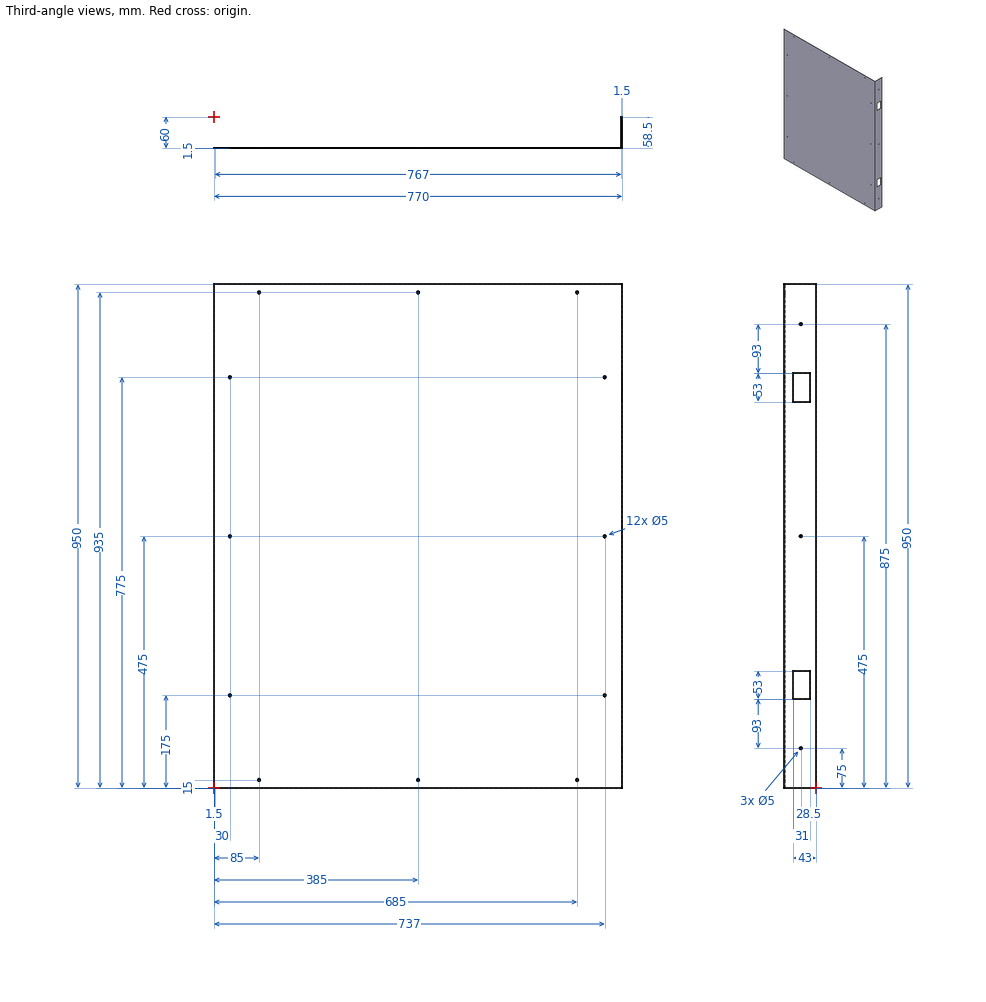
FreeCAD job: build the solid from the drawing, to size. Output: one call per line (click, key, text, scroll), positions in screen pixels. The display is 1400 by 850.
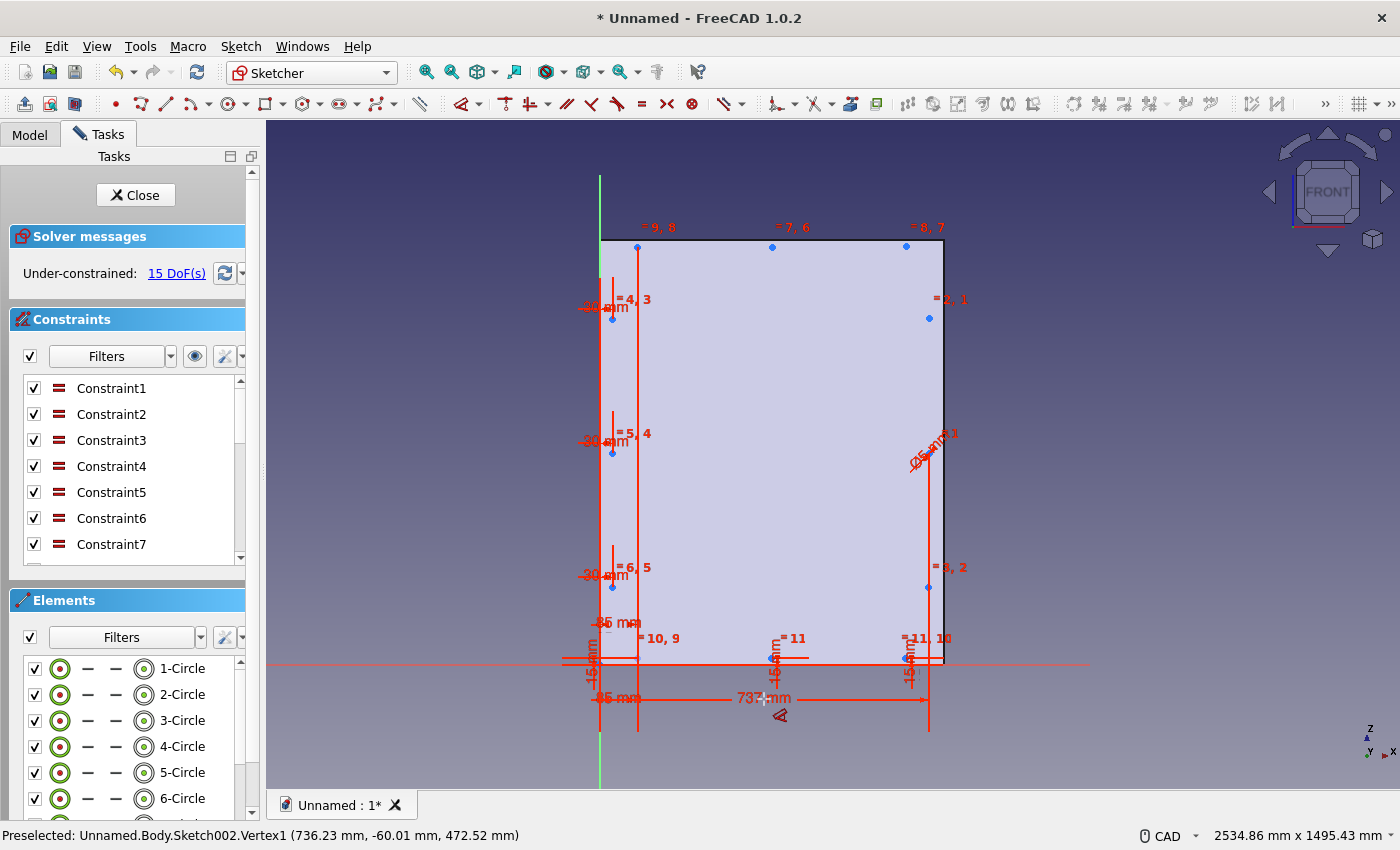
click(929, 453)
click(566, 510)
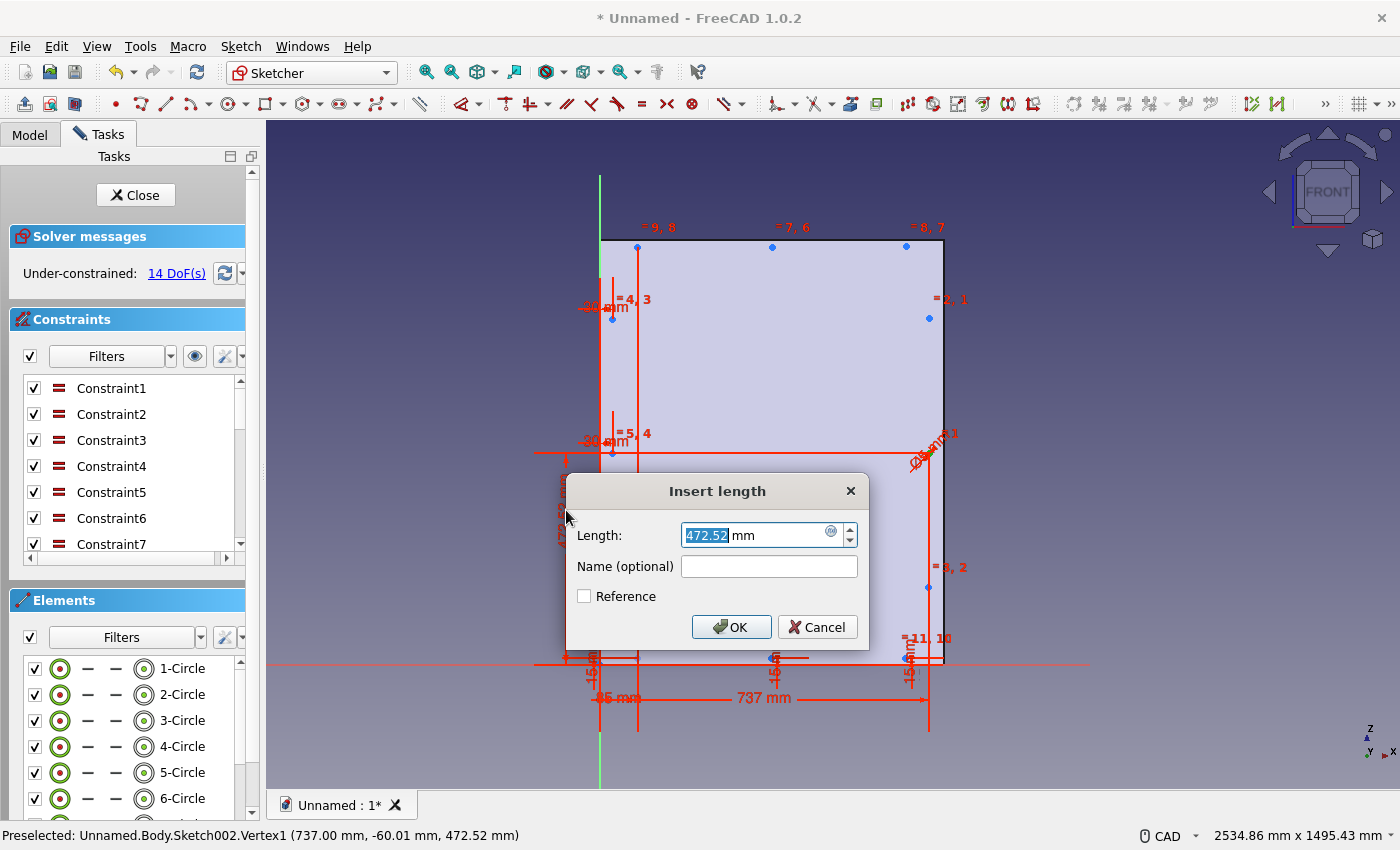
text(475)
key(Return)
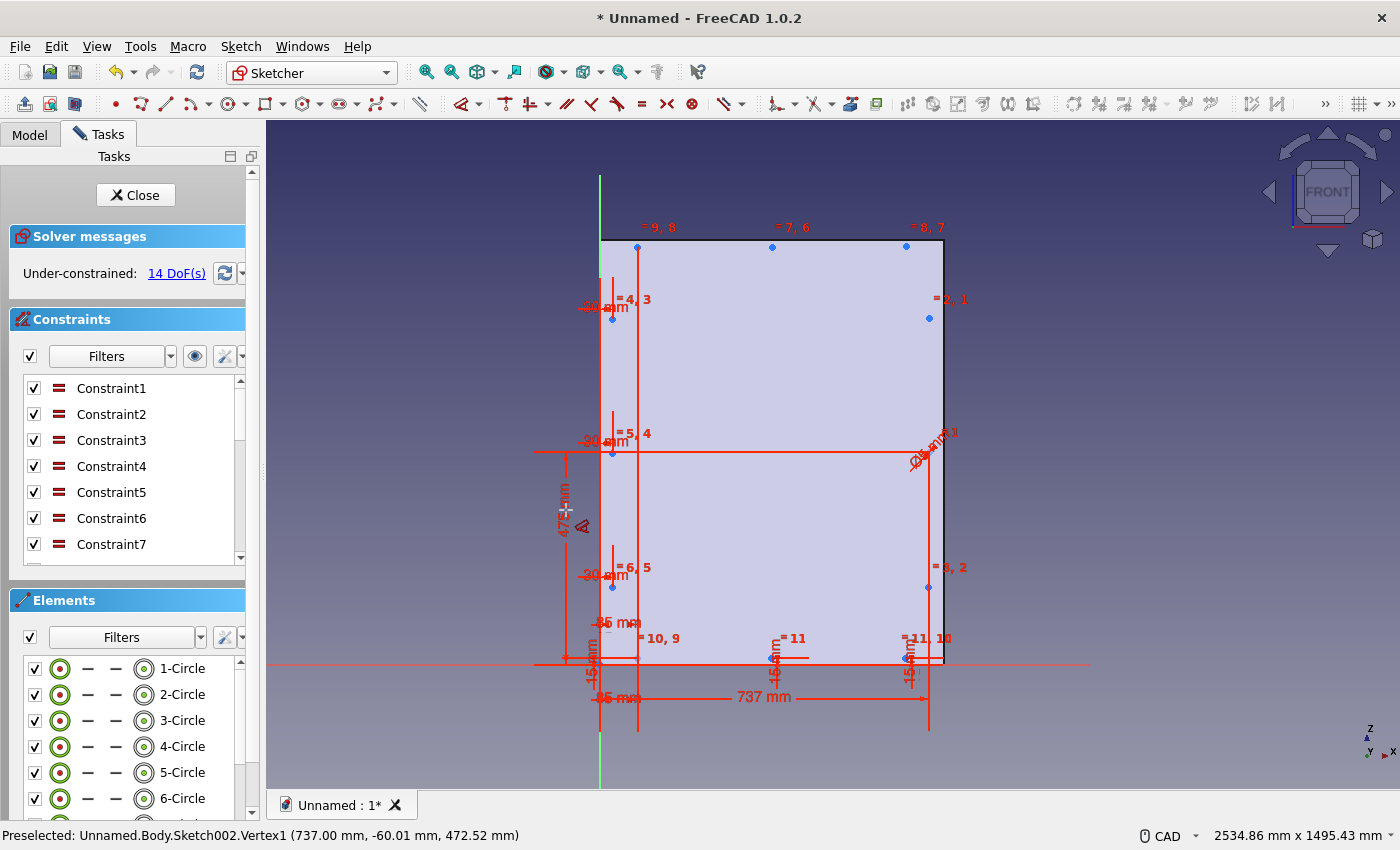
click(929, 319)
click(840, 699)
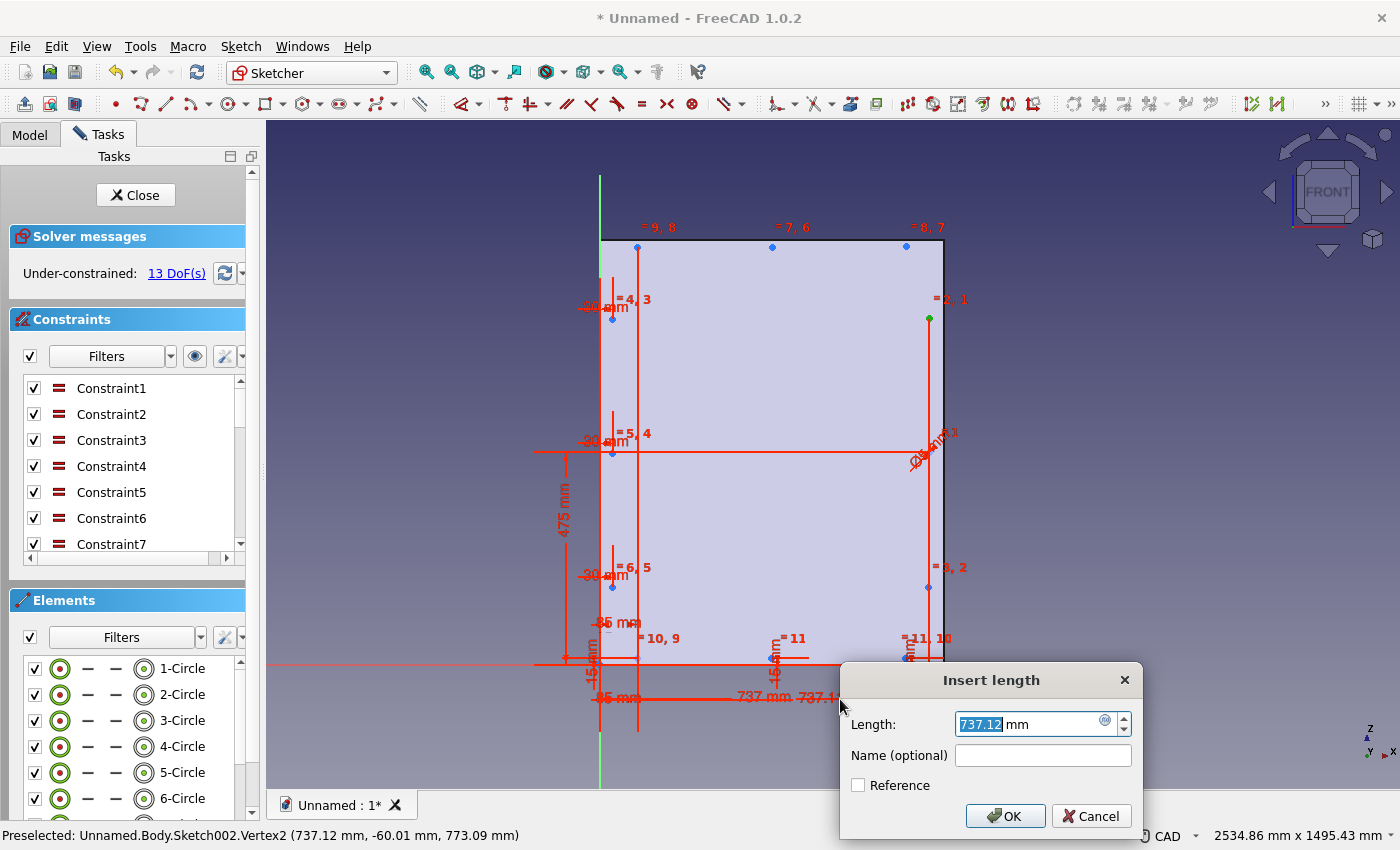
text(737)
key(Return)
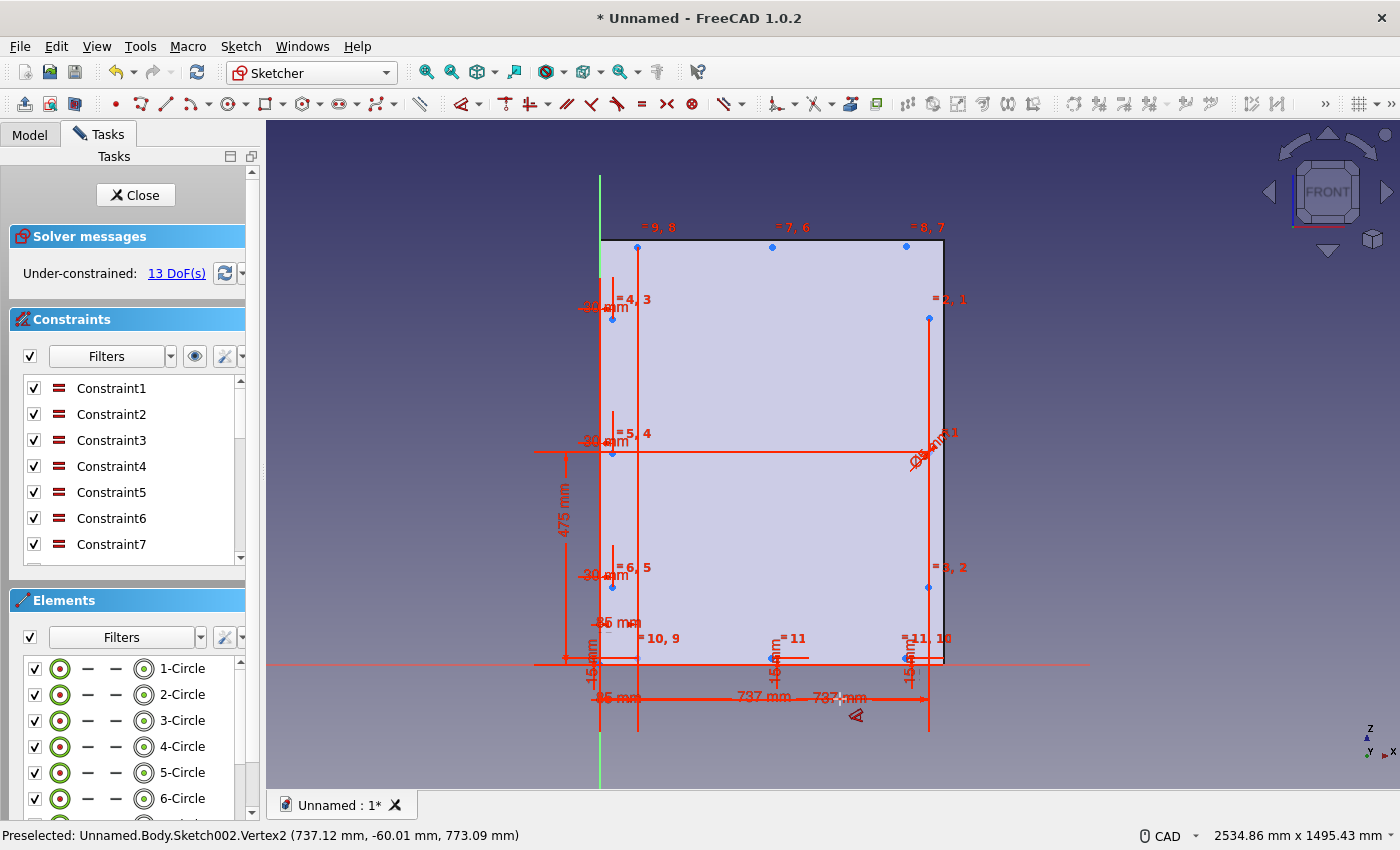
click(929, 319)
click(566, 412)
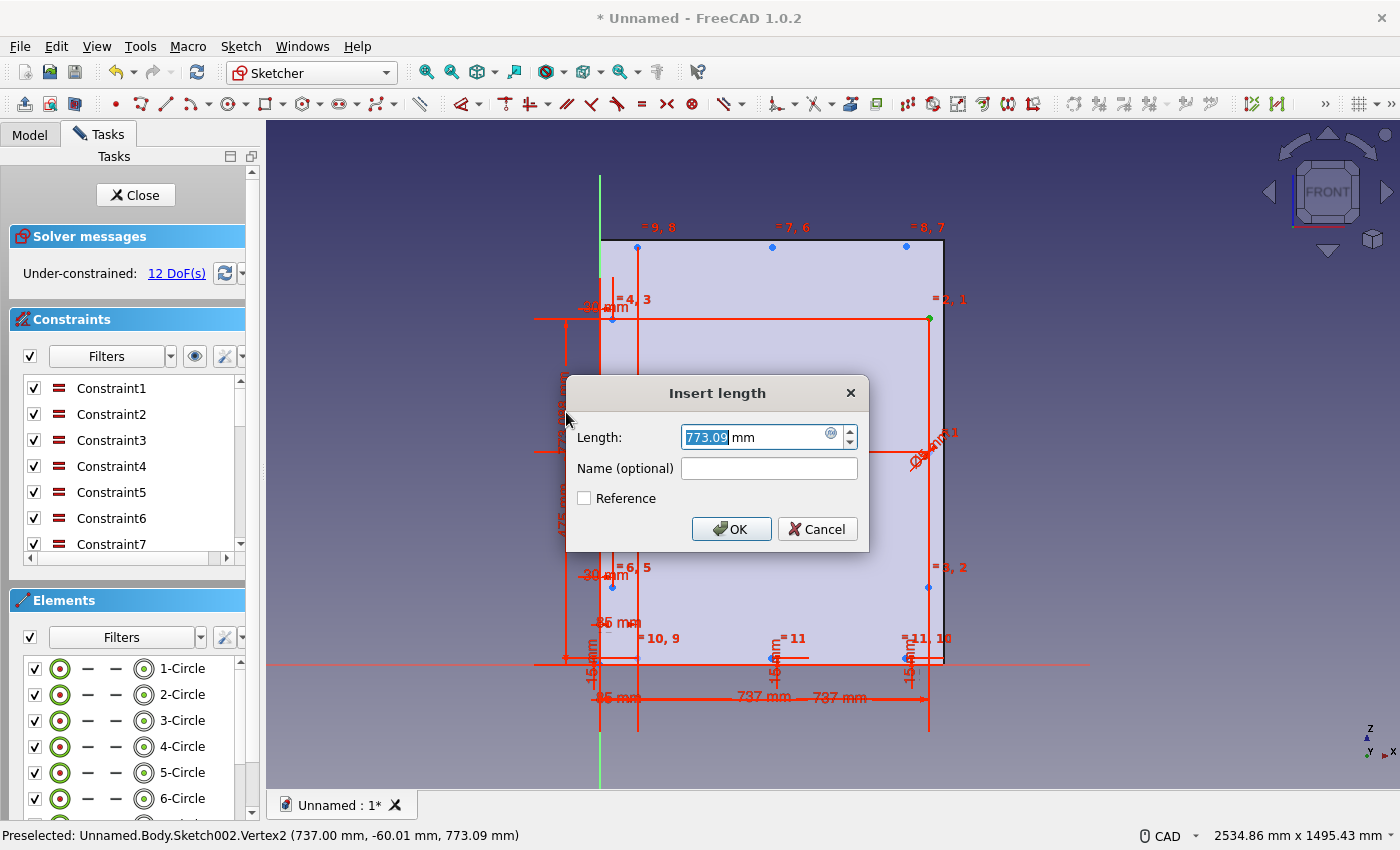
text(775)
key(Return)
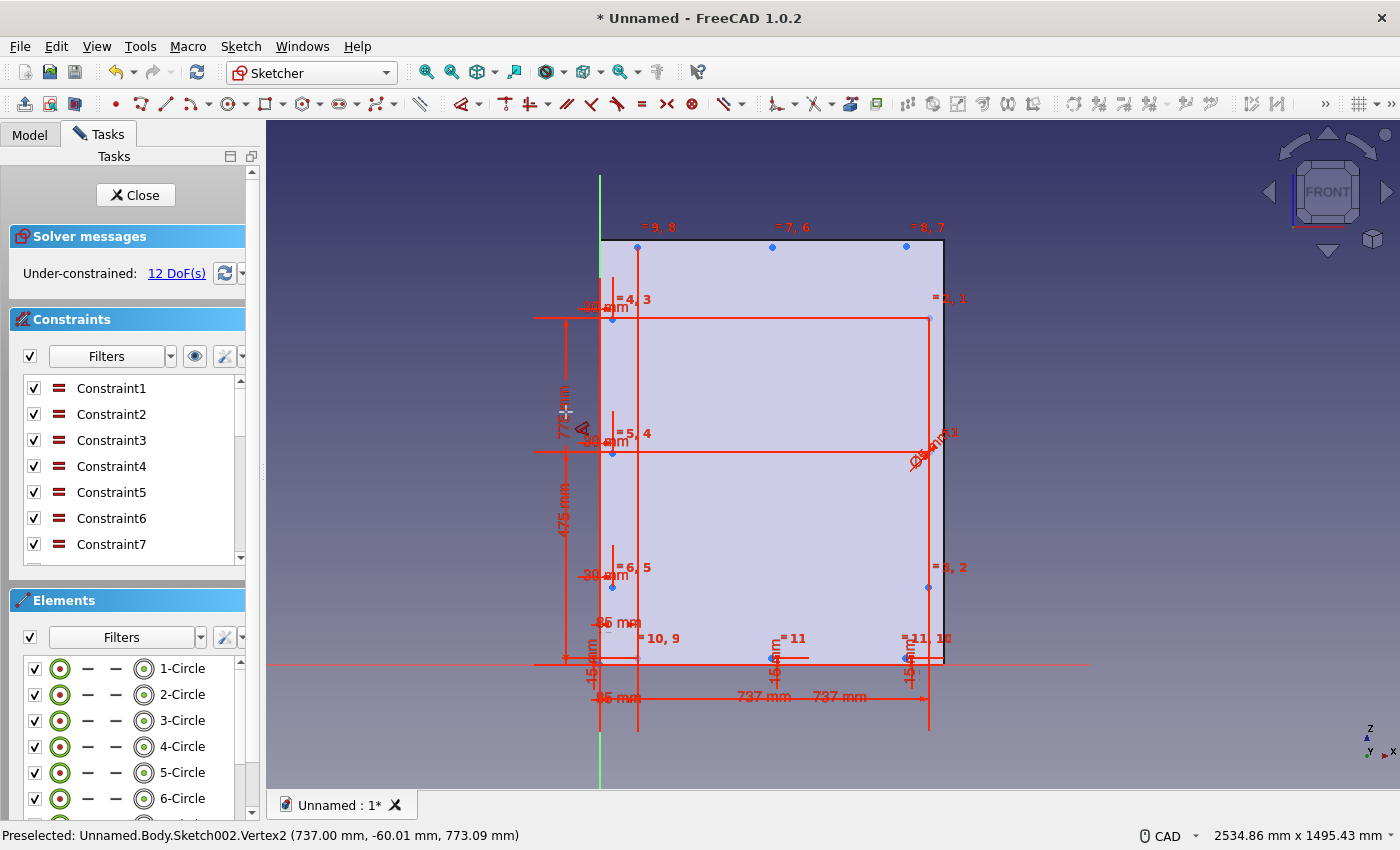
click(929, 588)
click(764, 554)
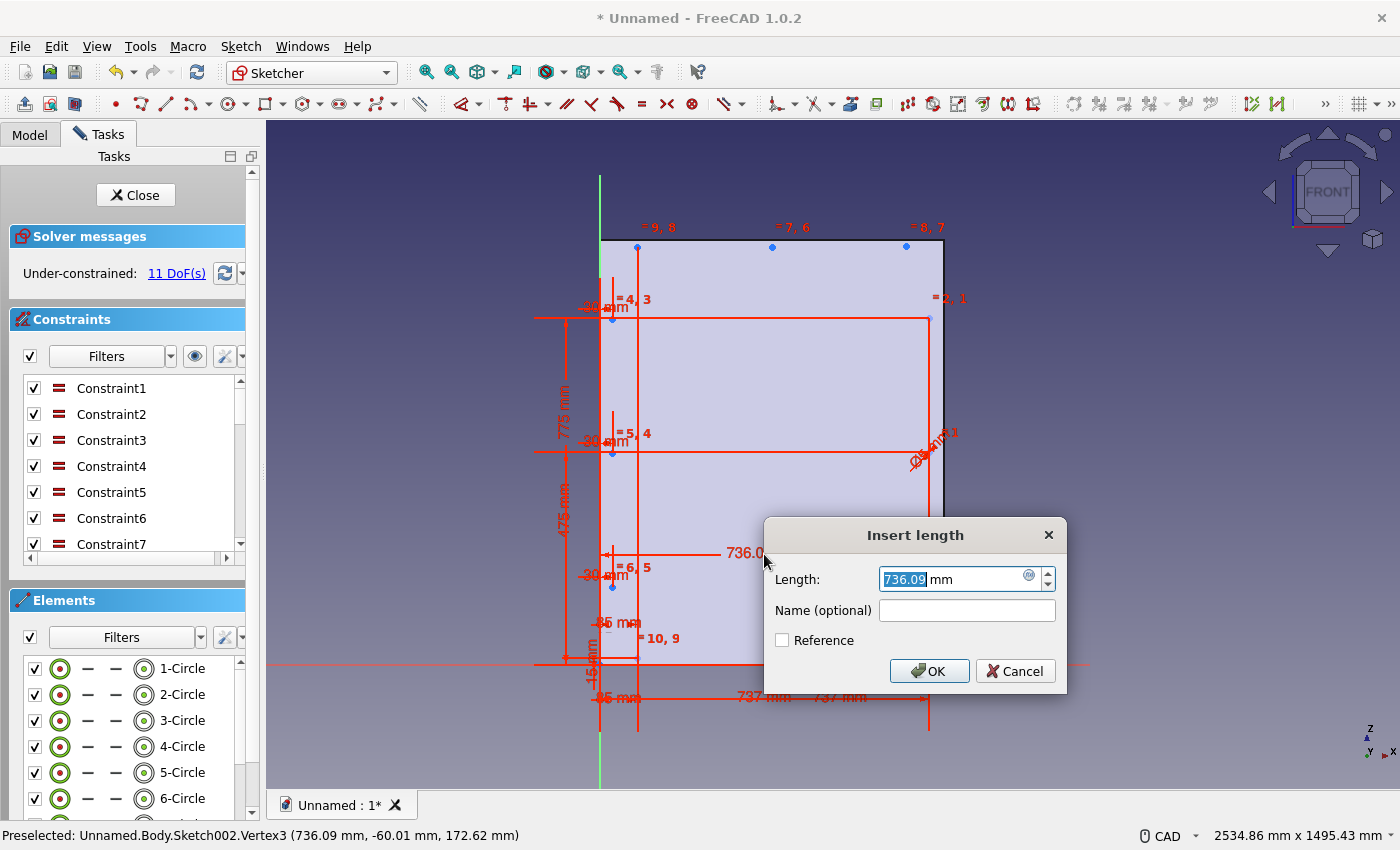
text(737)
key(Return)